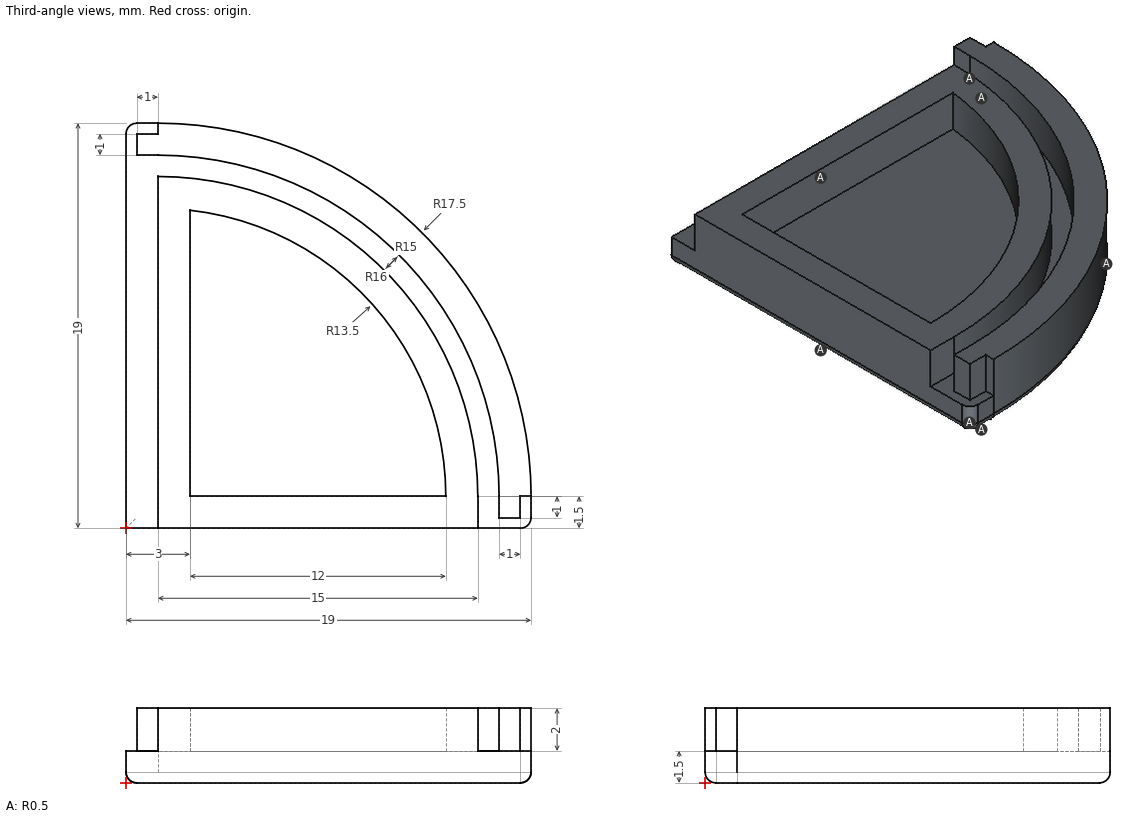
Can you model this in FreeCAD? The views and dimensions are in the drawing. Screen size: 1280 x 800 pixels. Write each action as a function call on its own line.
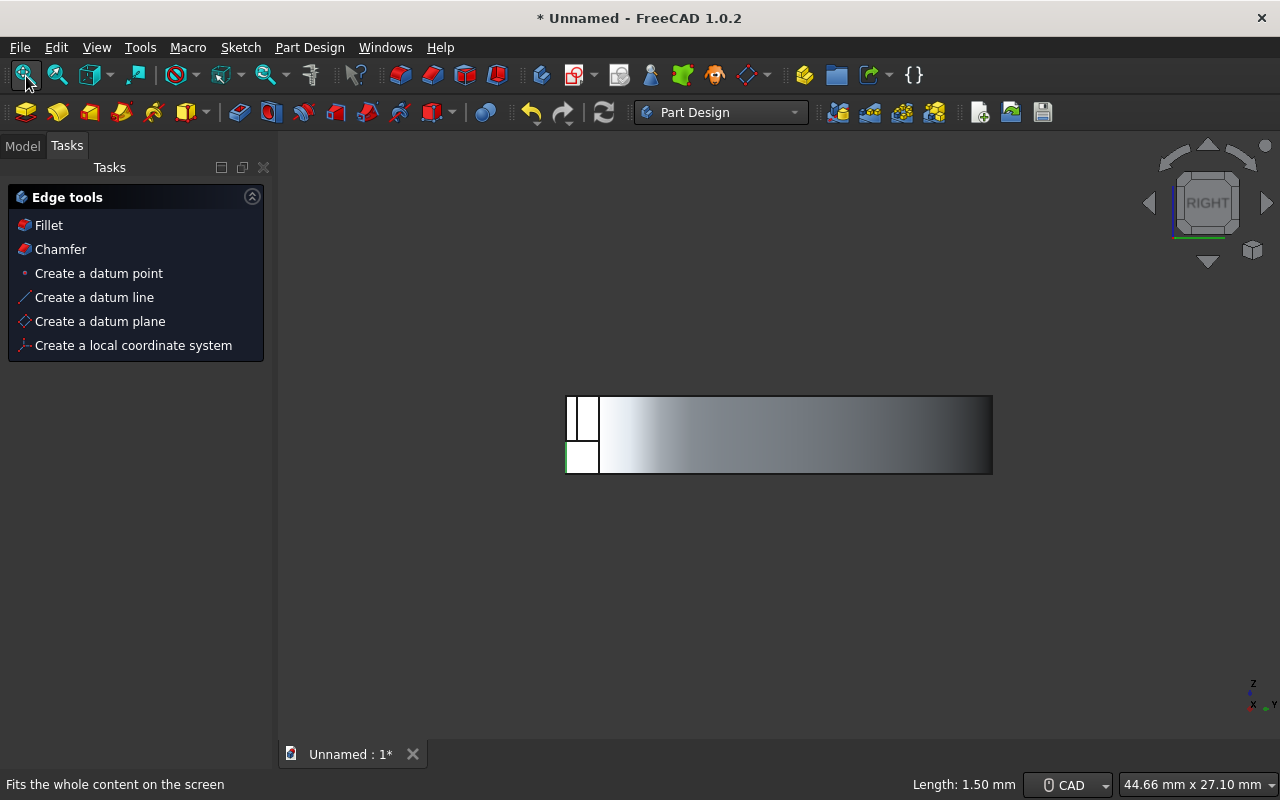
key(v)
key(f)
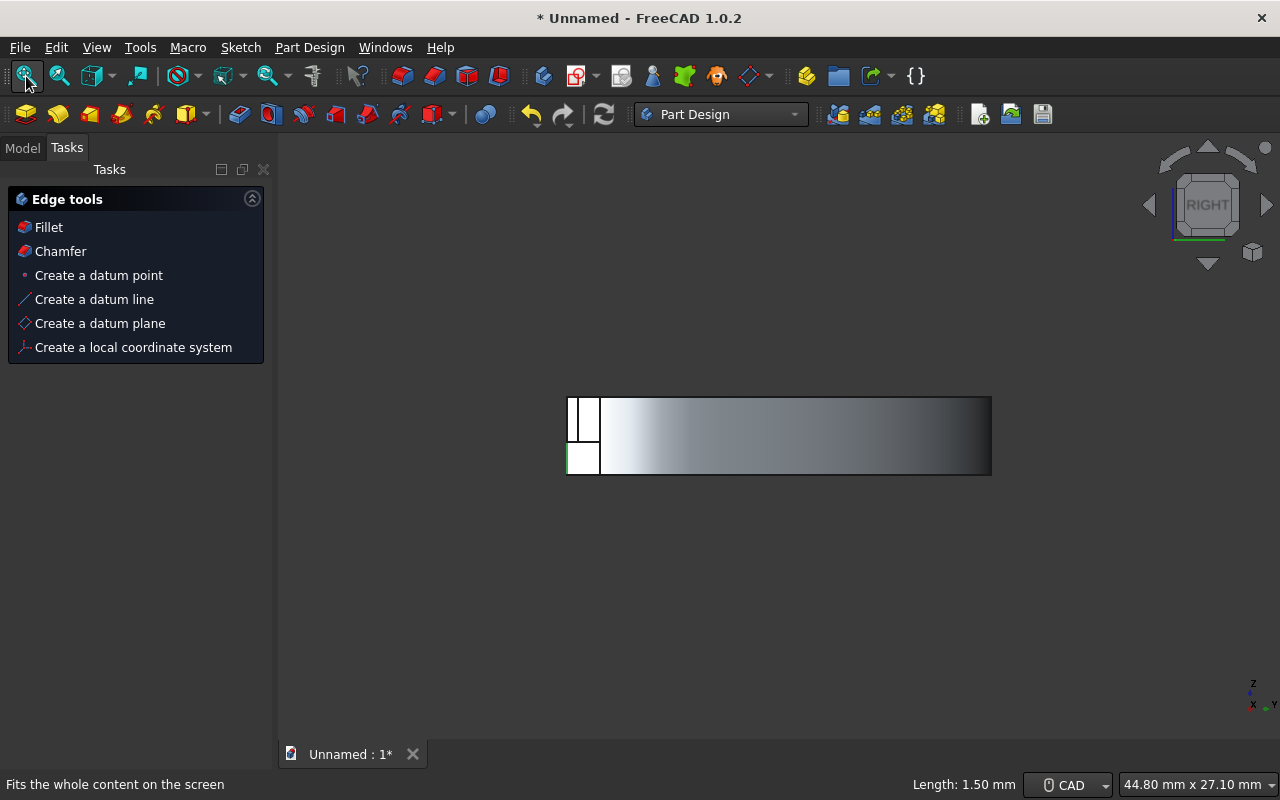
key(5)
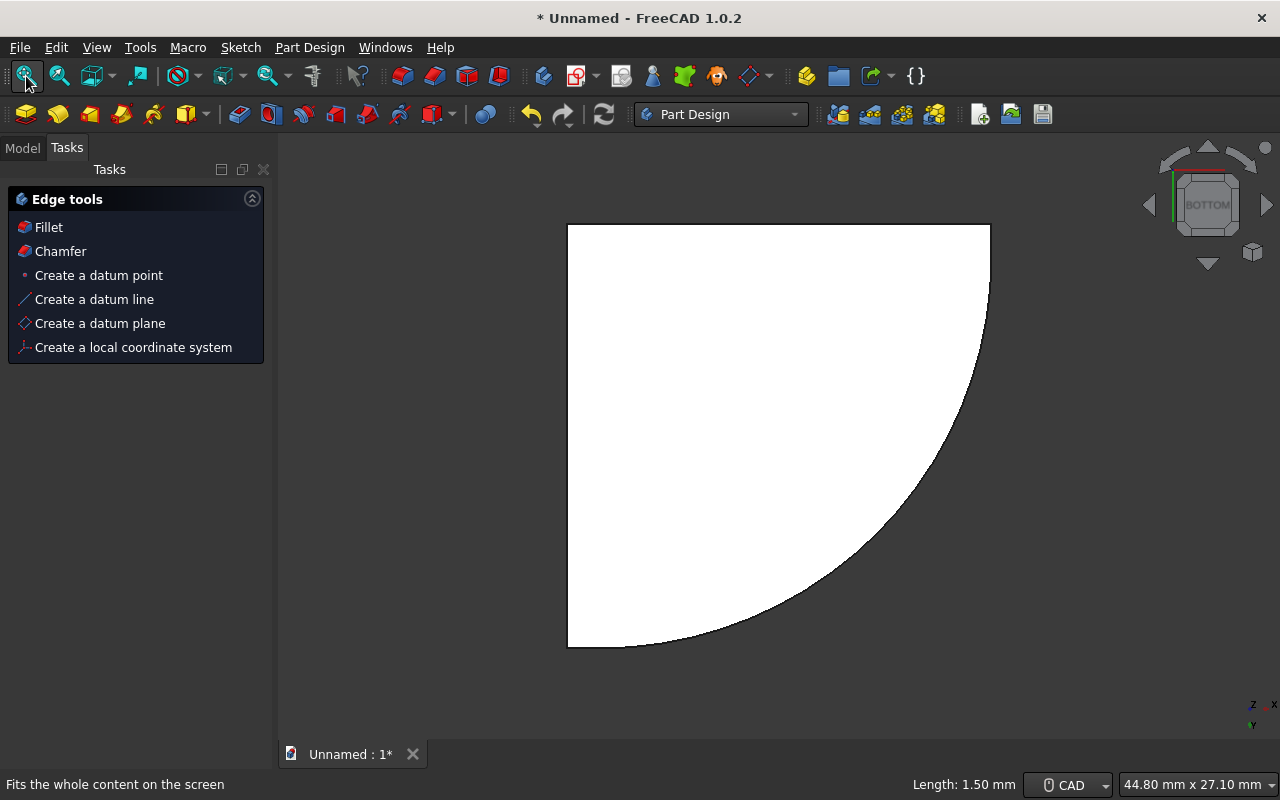
click(779, 374, ctrl)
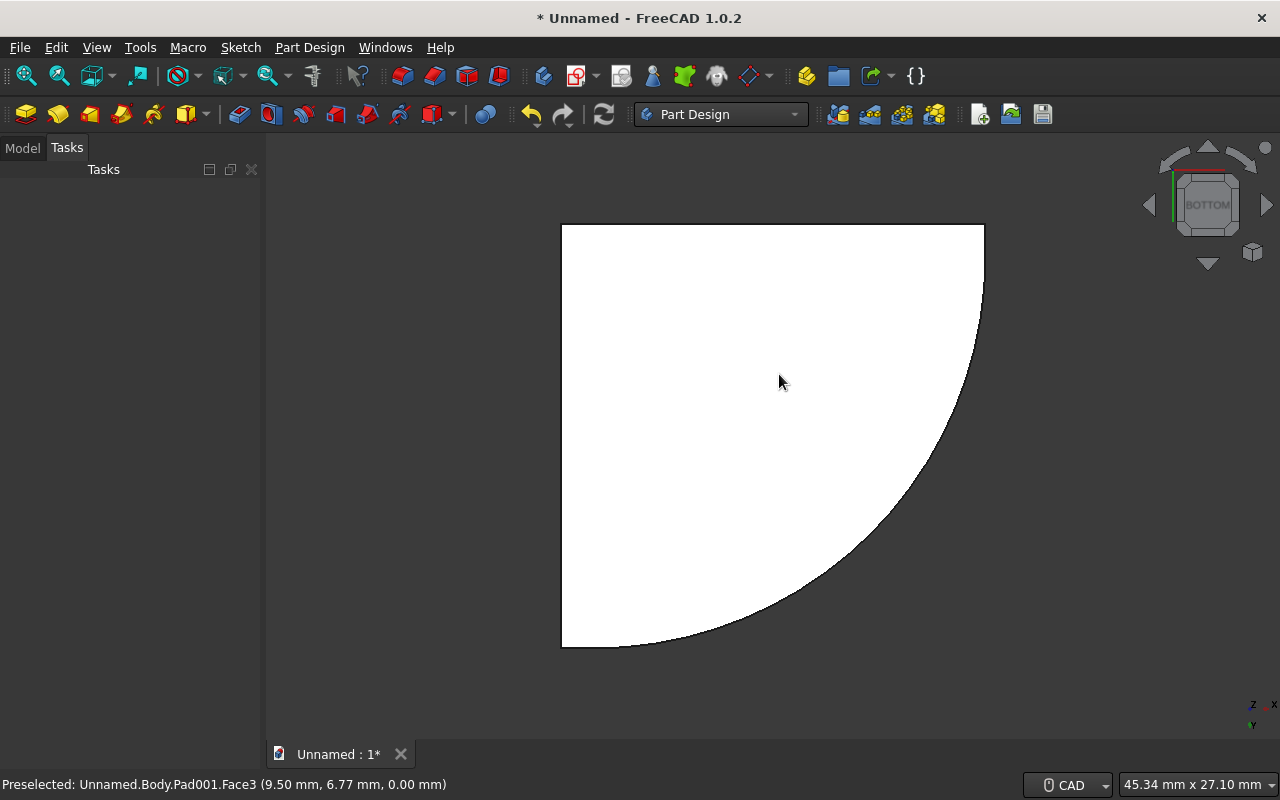
key(4)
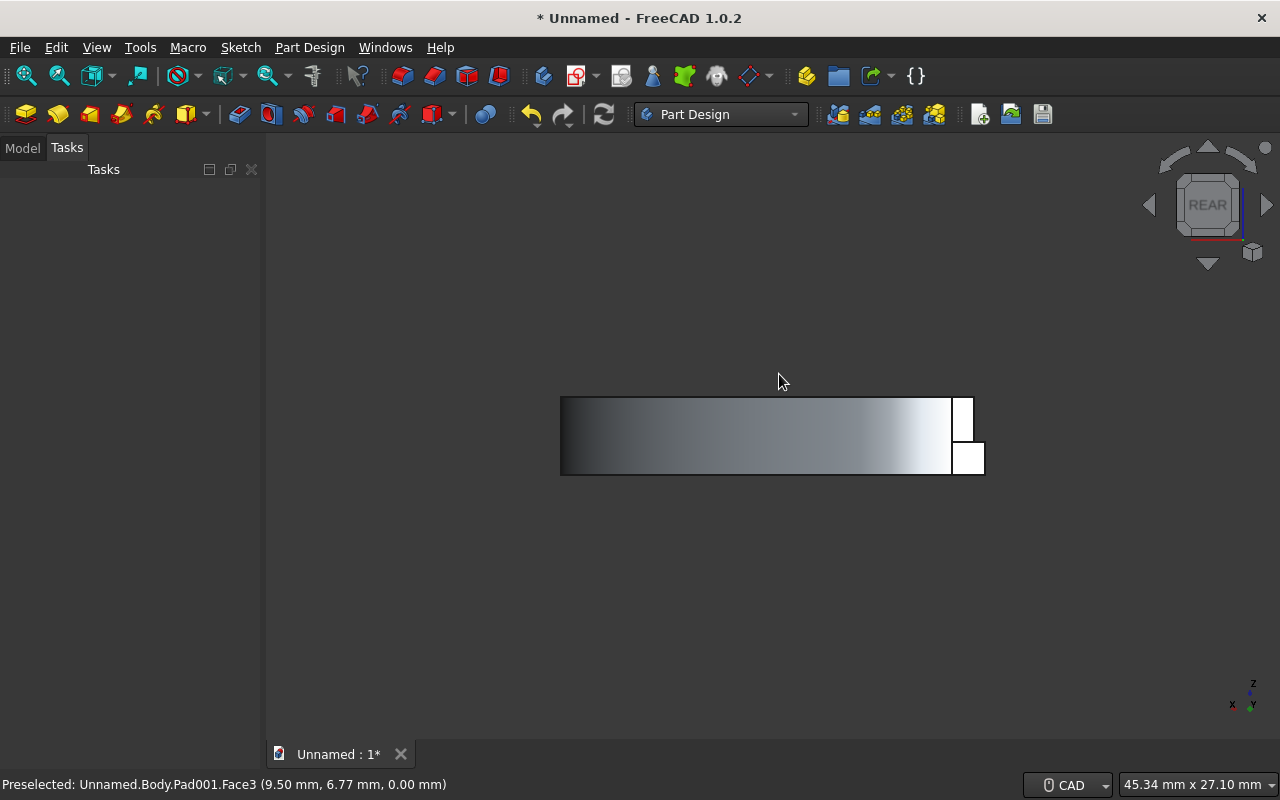
click(28, 76)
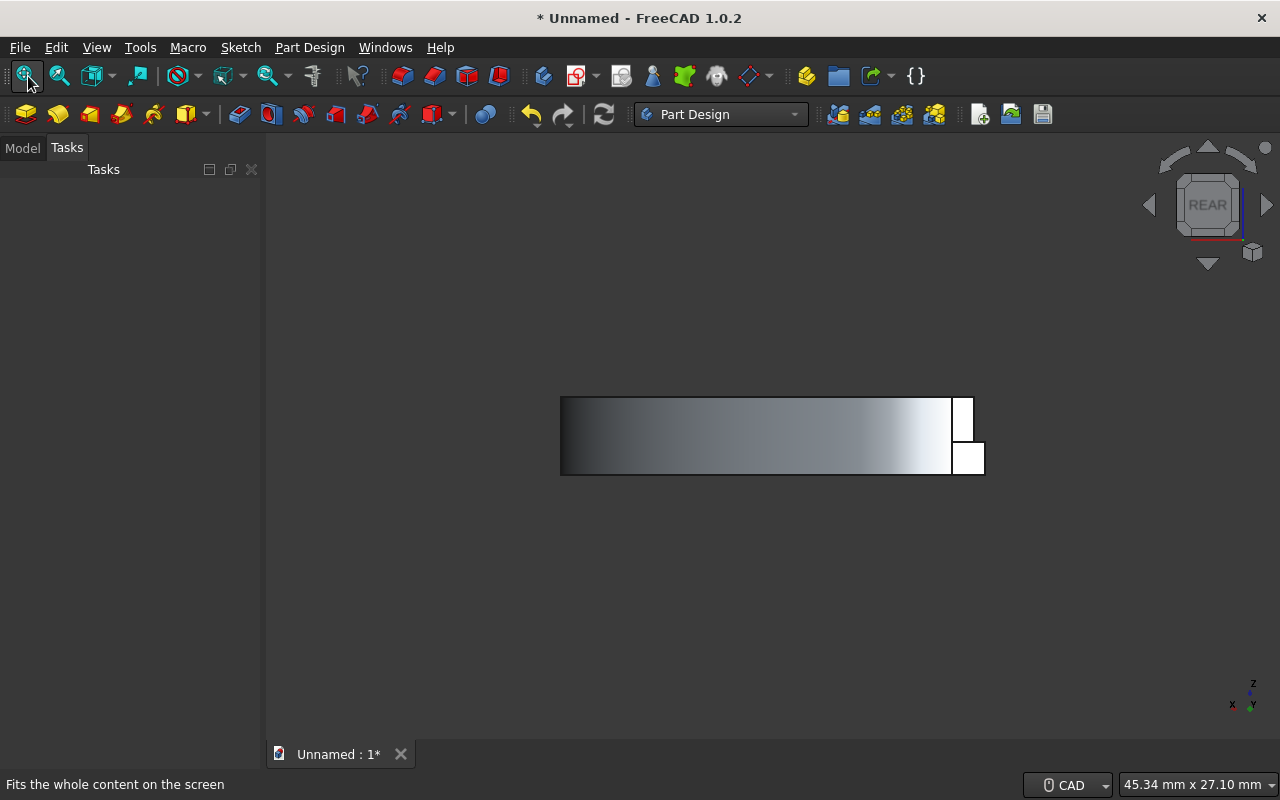
click(985, 457, ctrl)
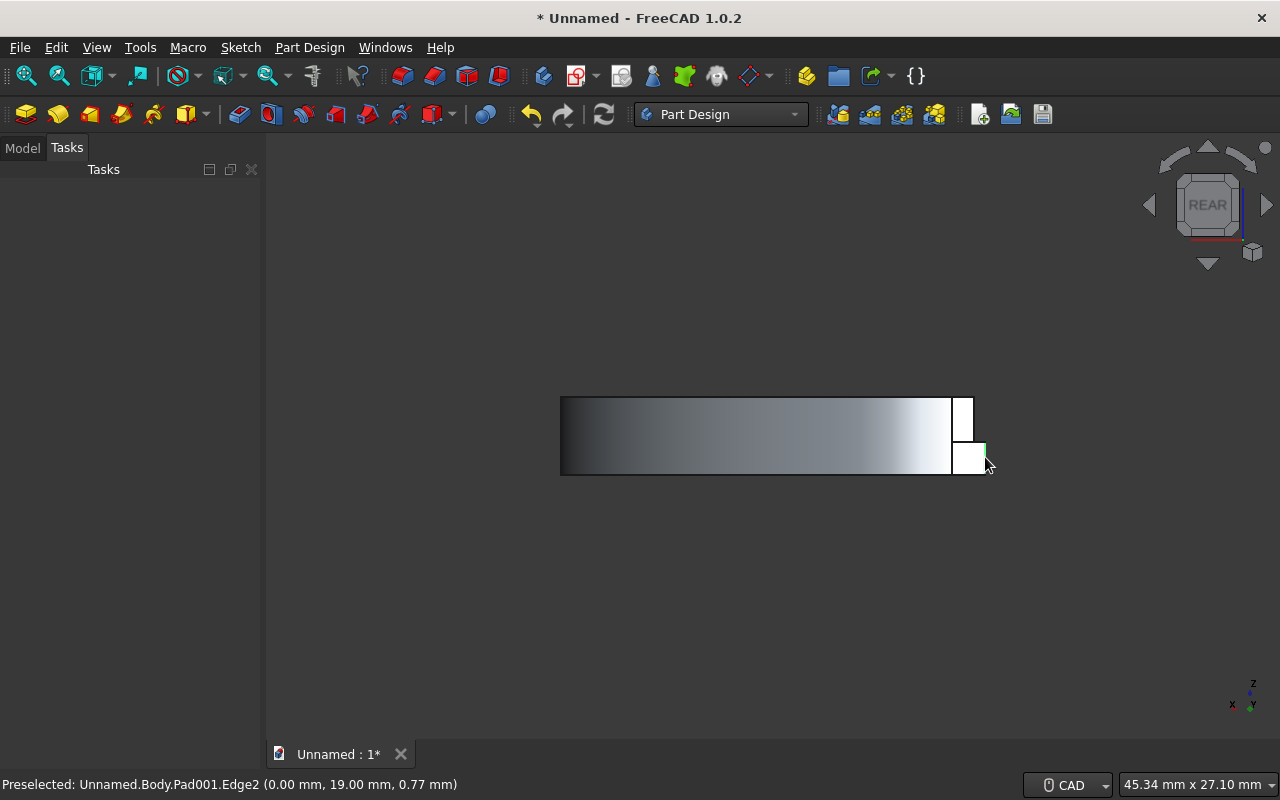
click(404, 76)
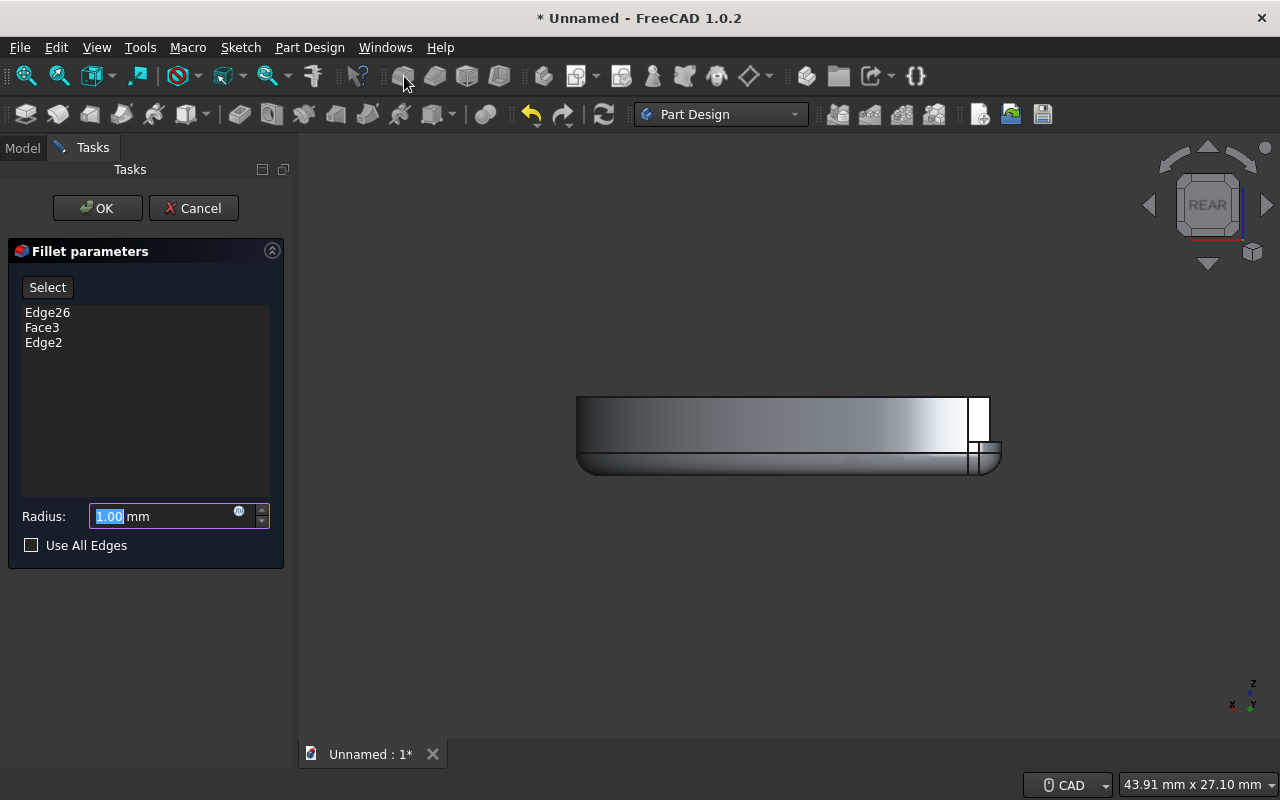
text(0.5)
key(Tab)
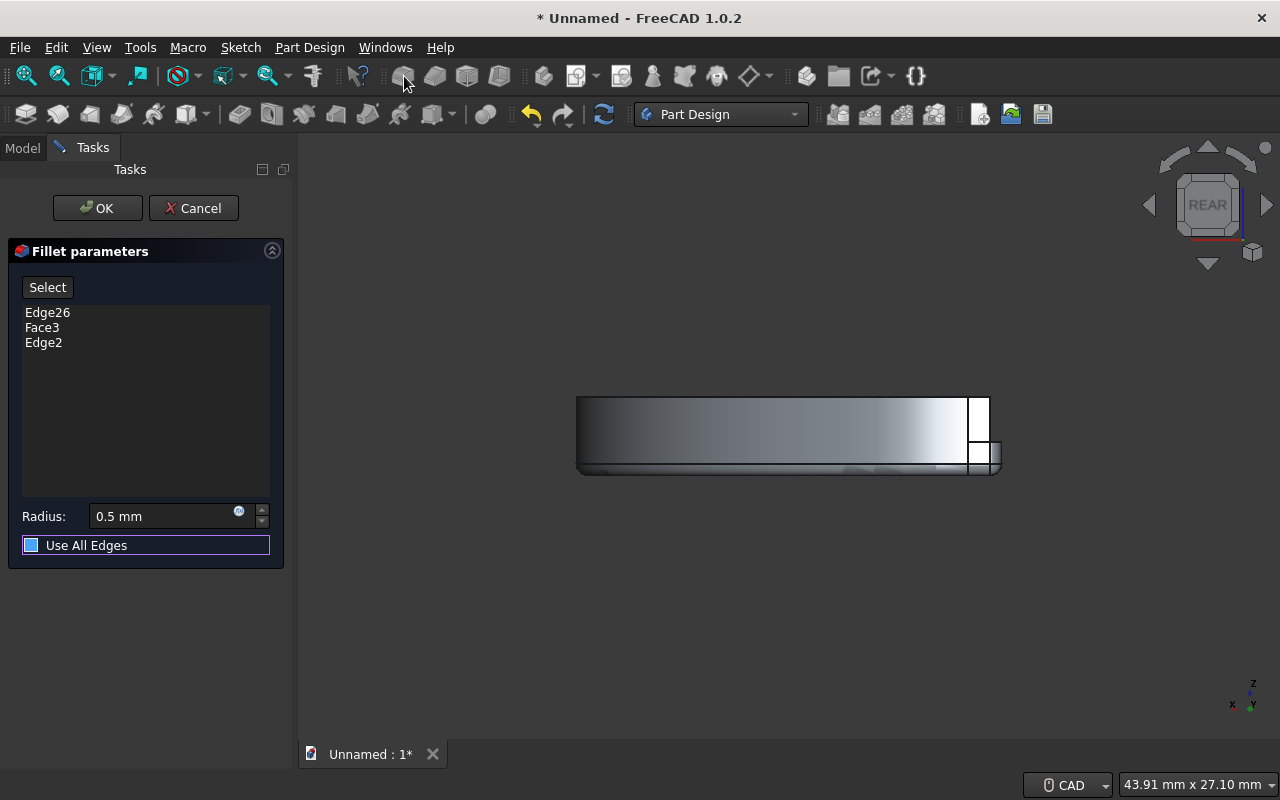
click(98, 208)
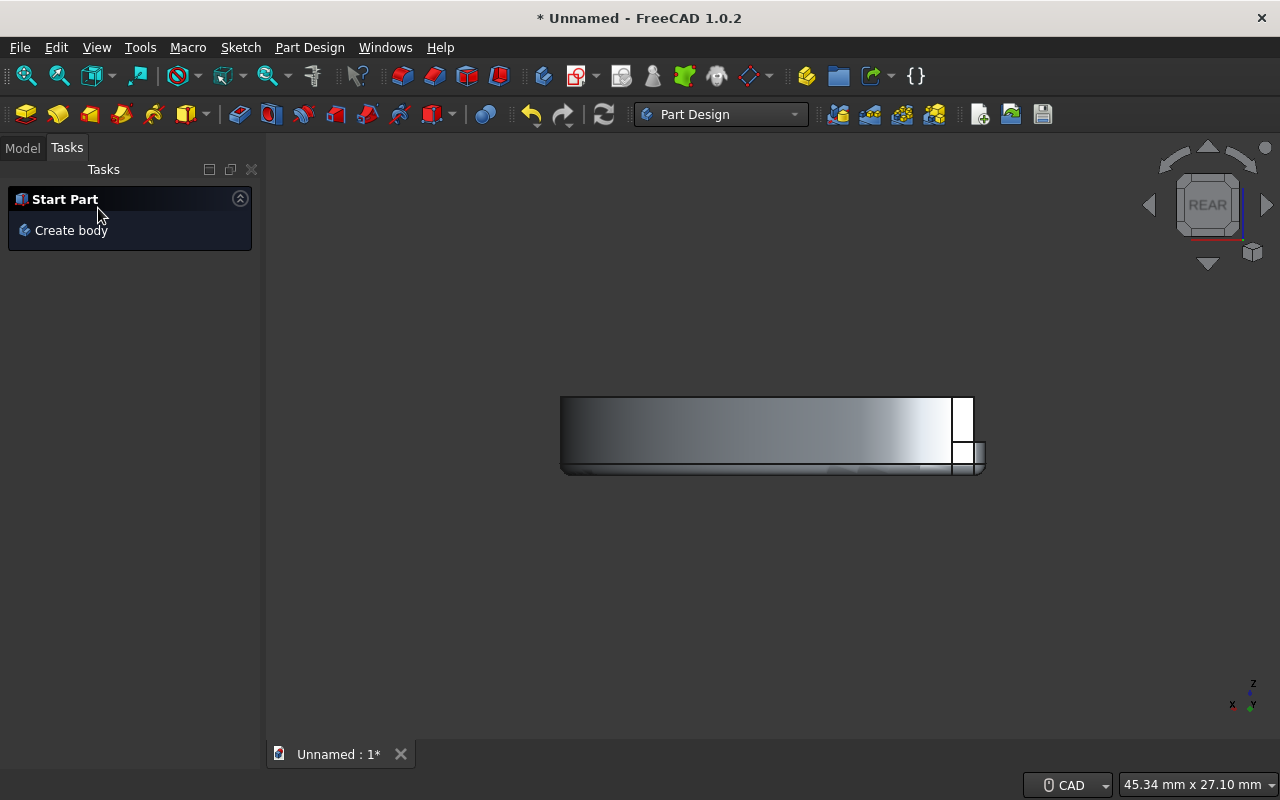
key(0)